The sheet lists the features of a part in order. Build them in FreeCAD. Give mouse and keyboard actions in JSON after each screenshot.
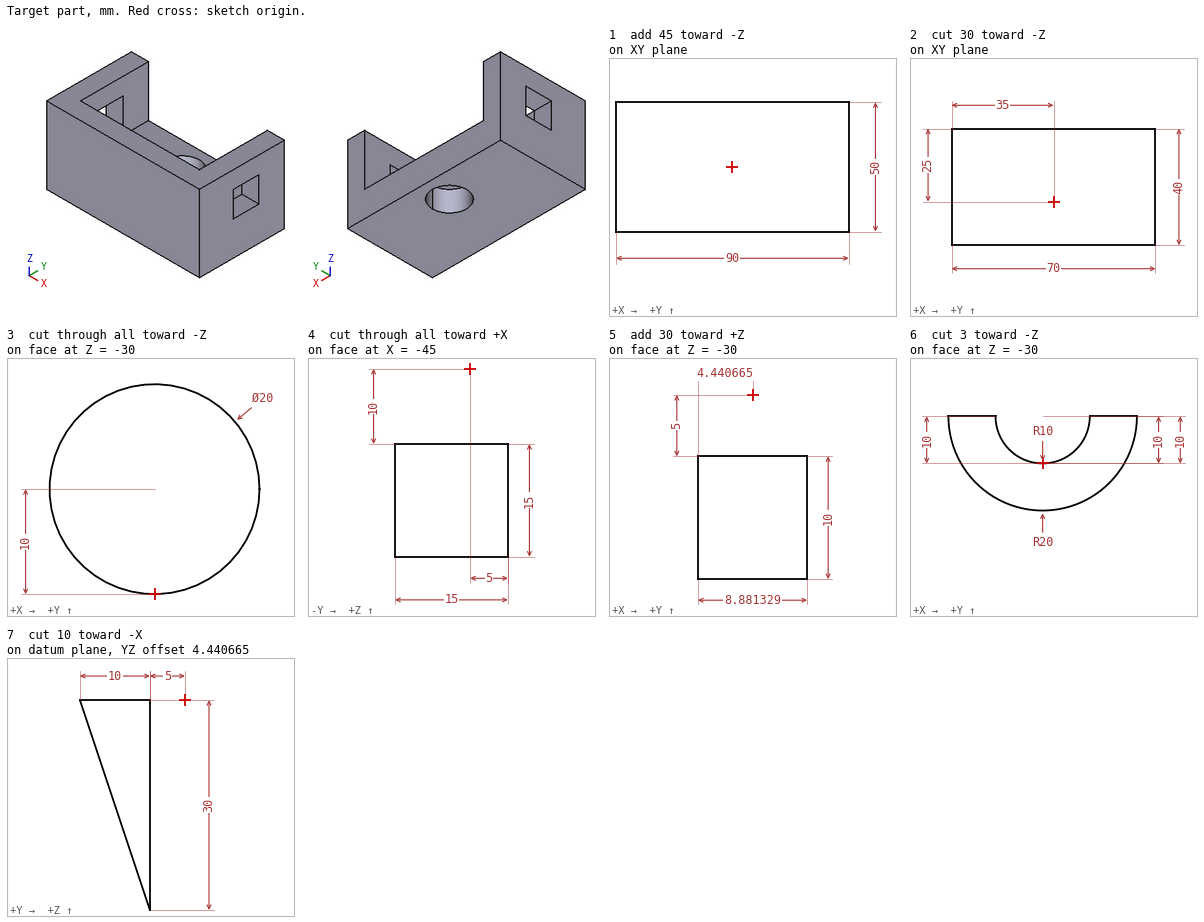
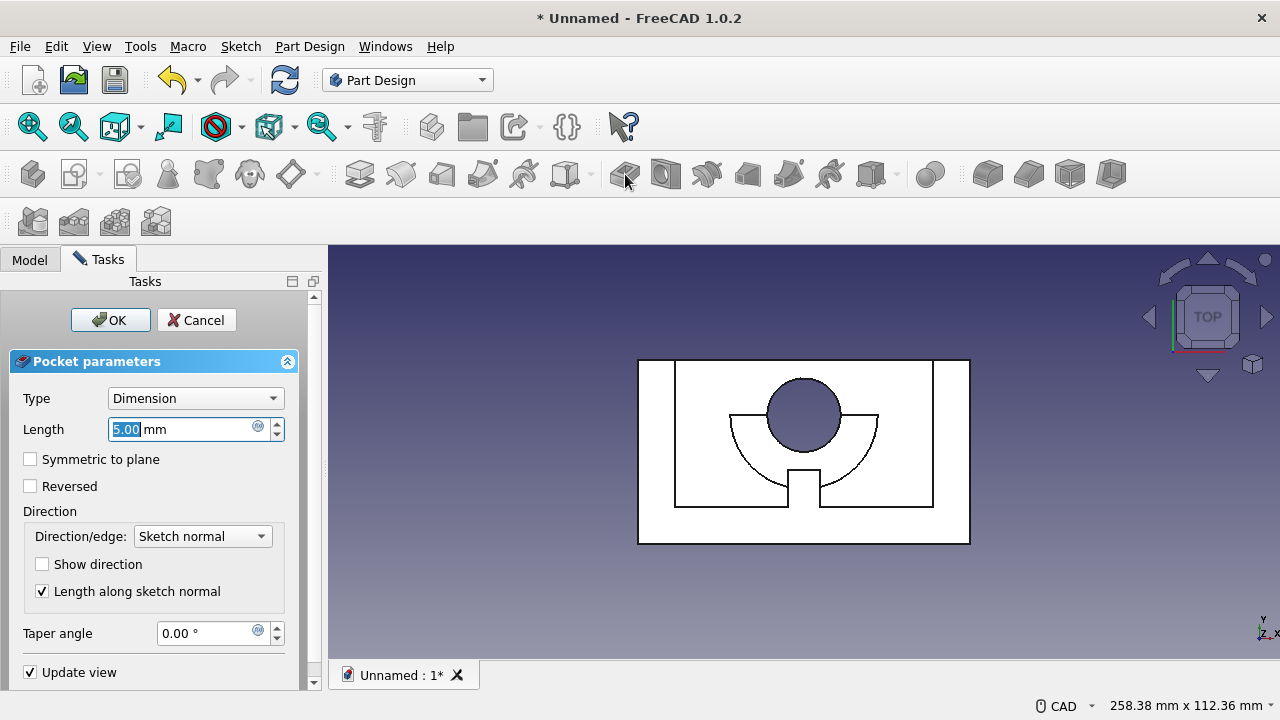
{"action": "type", "text": "3"}
{"action": "key", "text": "Tab"}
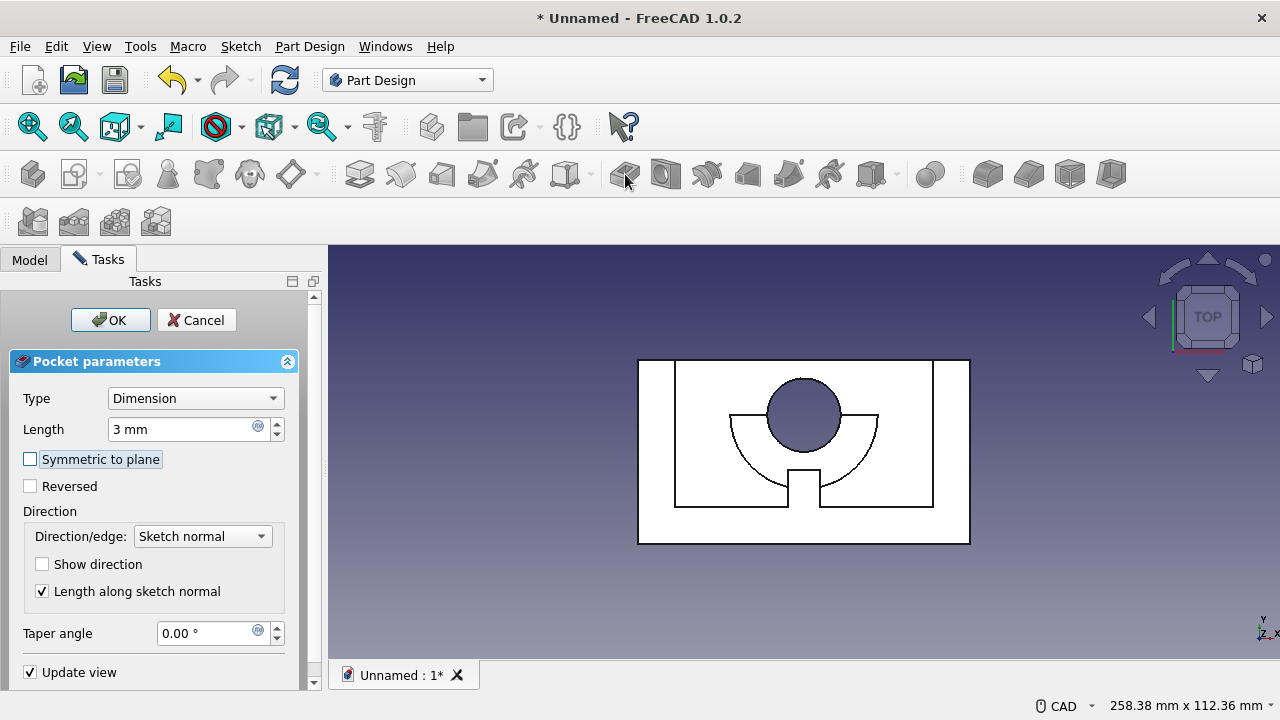
{"action": "left_click", "coordinate": [111, 320]}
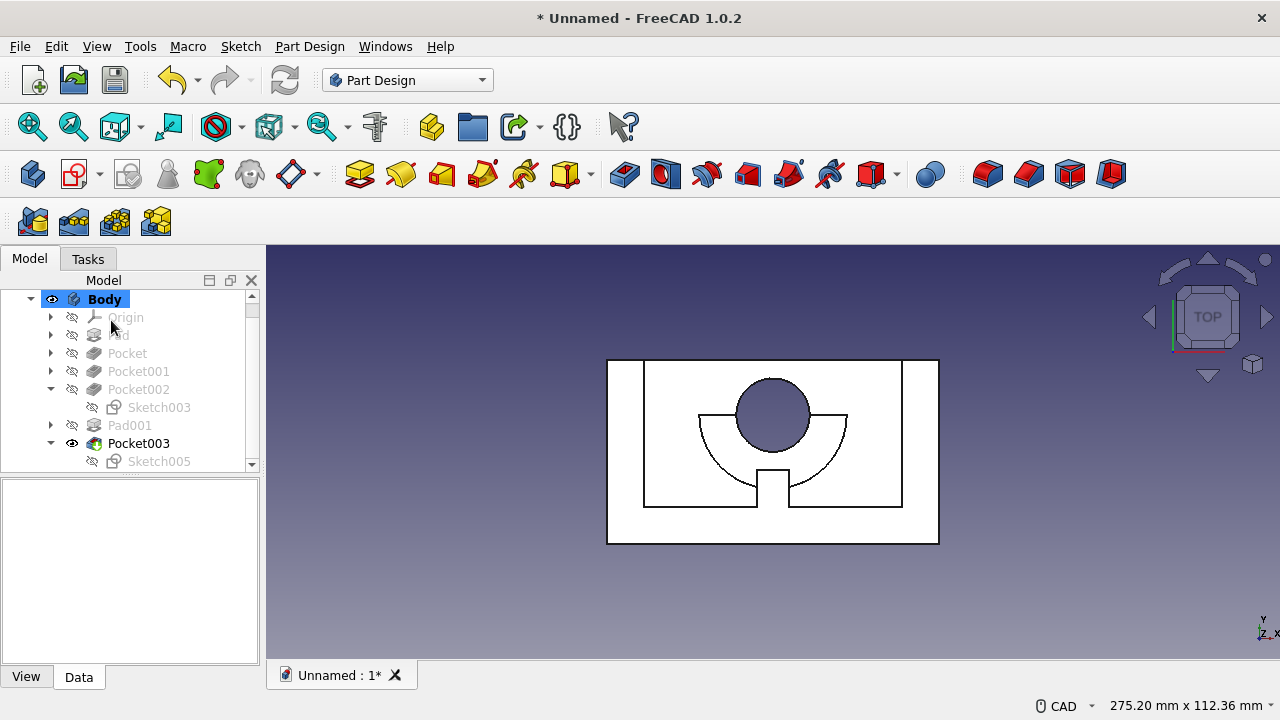
{"action": "left_click", "coordinate": [33, 128]}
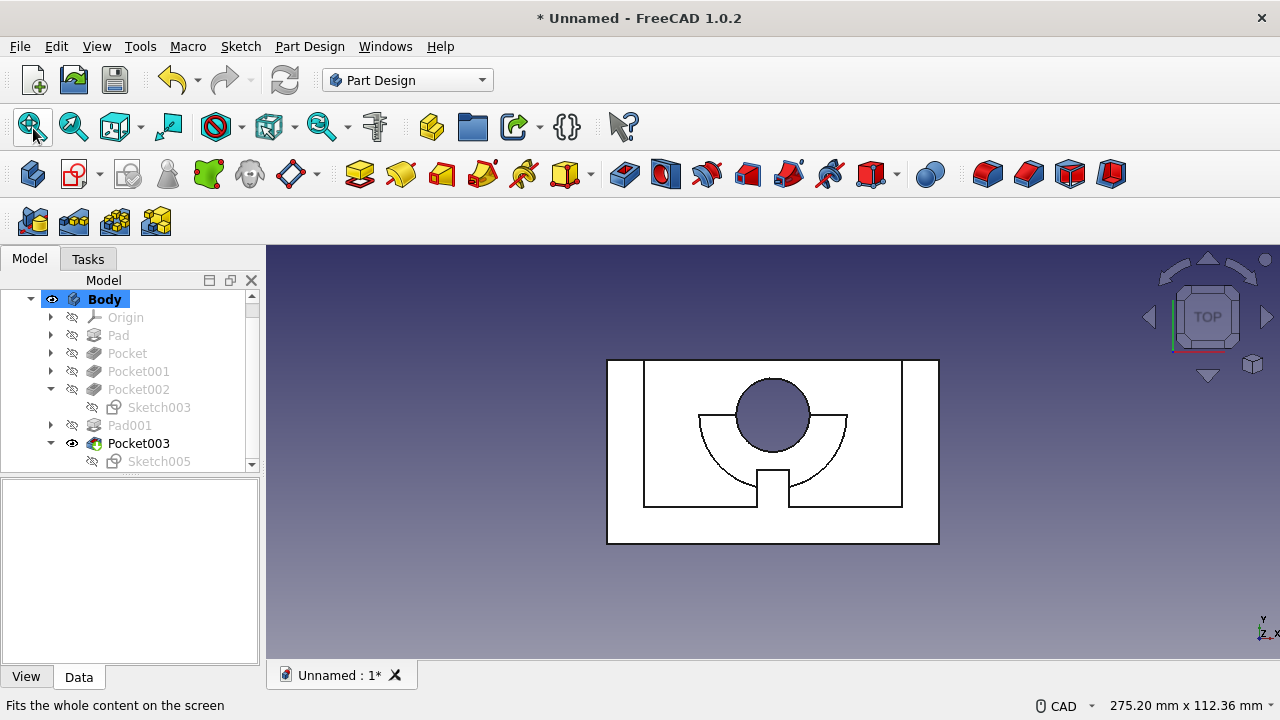
{"action": "left_click", "coordinate": [51, 317]}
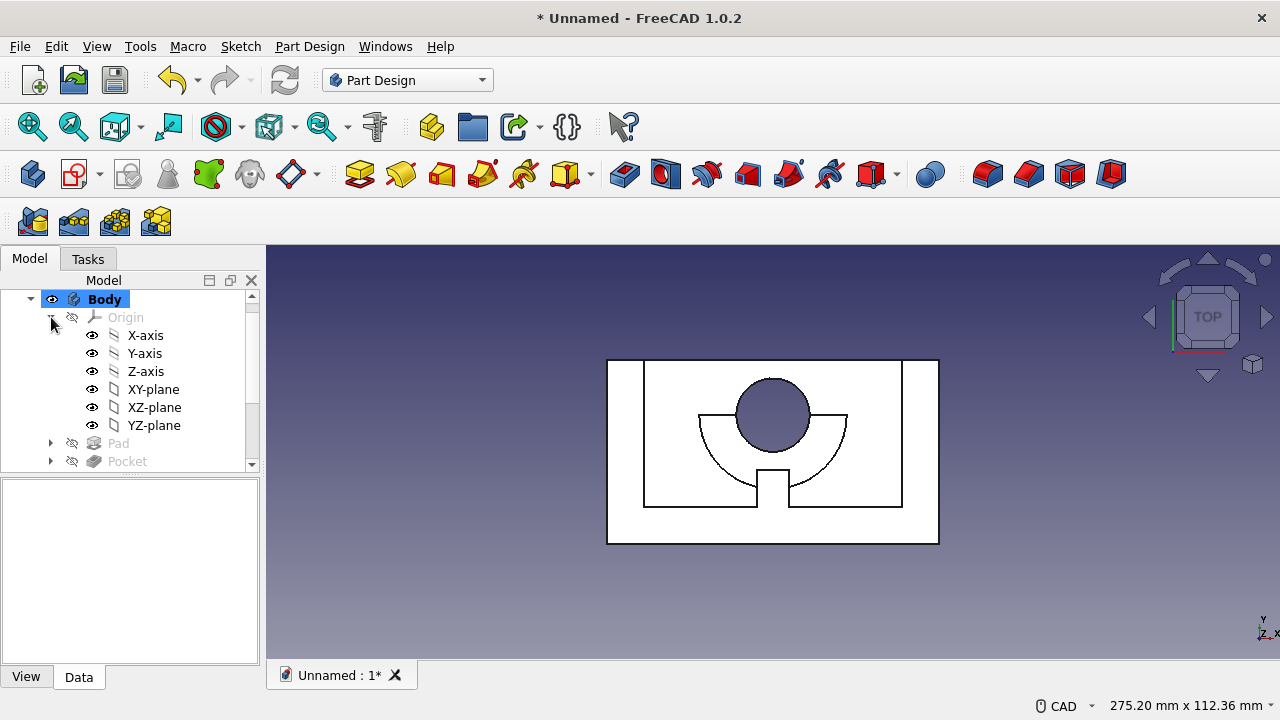
{"action": "left_click", "coordinate": [137, 425]}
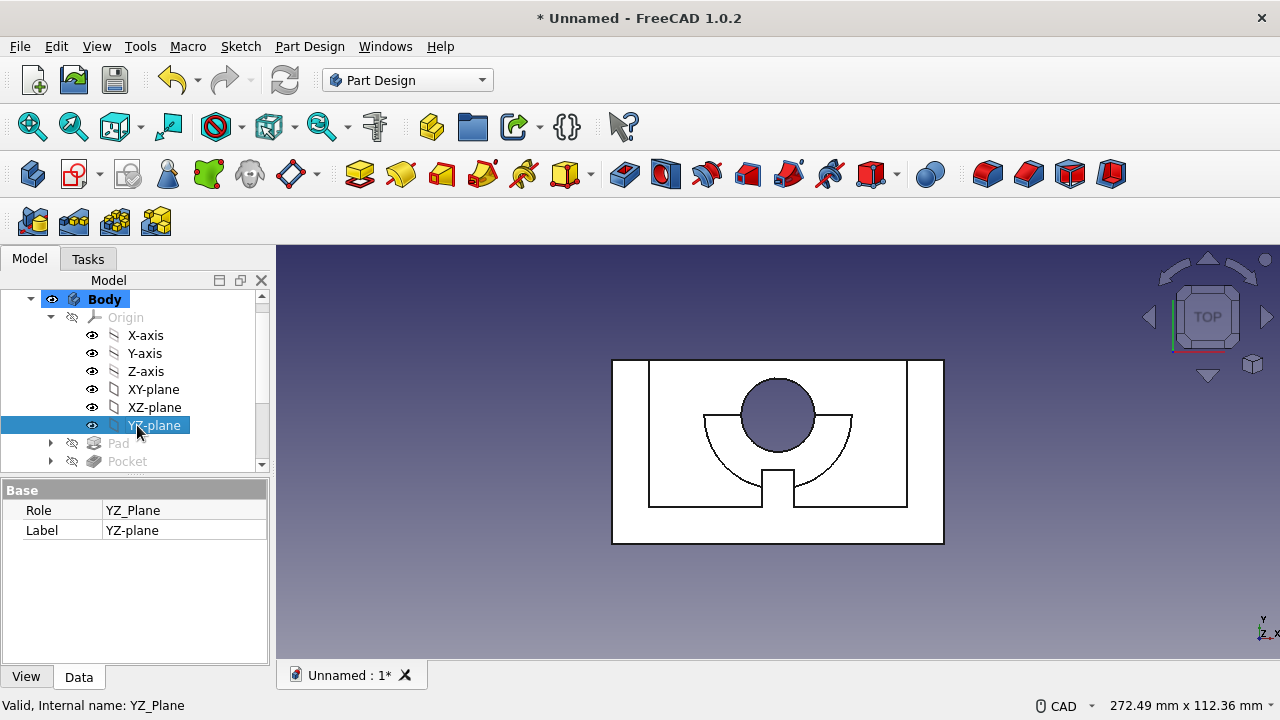
{"action": "left_click", "coordinate": [290, 174]}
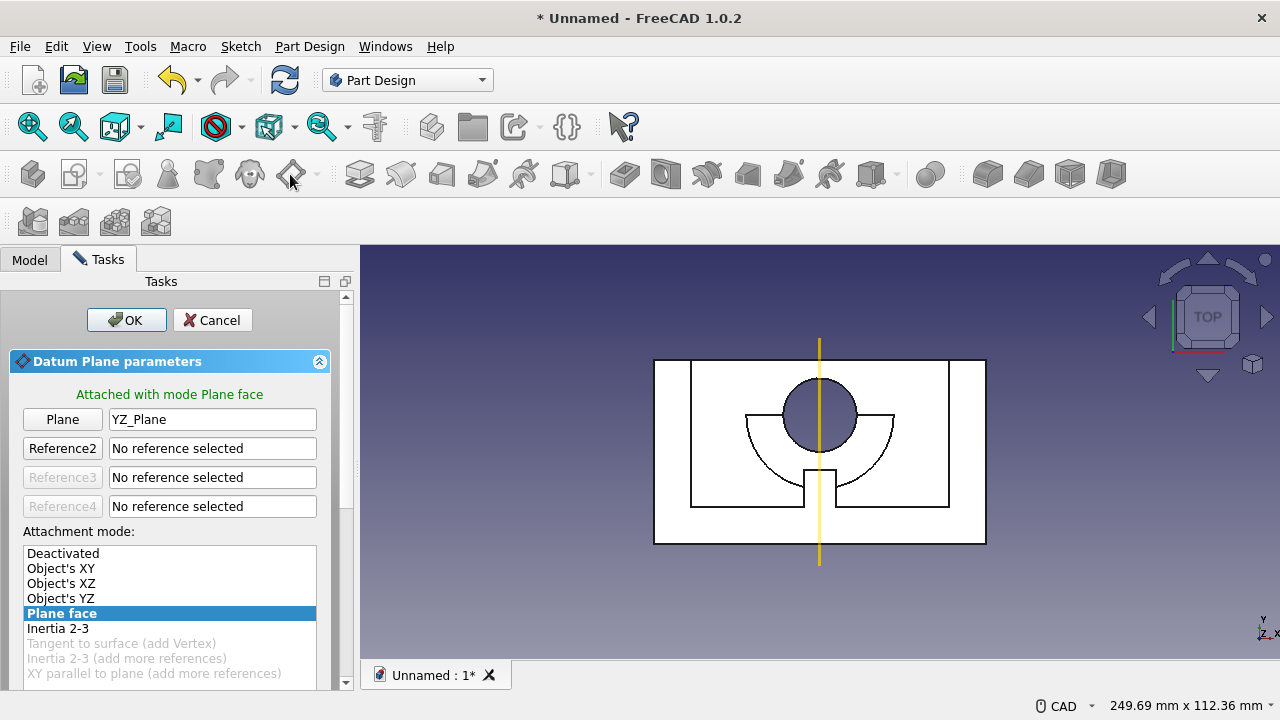
{"action": "scroll", "coordinate": [346, 490], "scroll_direction": "down", "scroll_amount": 4}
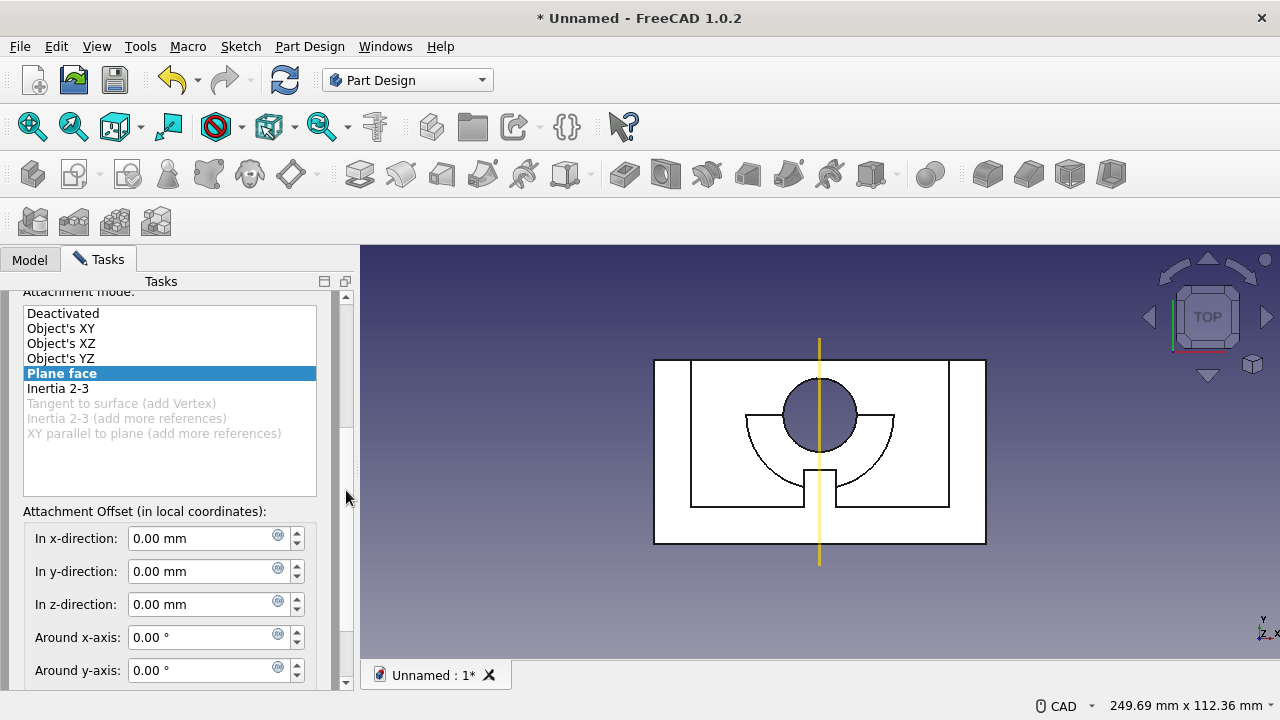
{"action": "triple_click", "coordinate": [210, 604]}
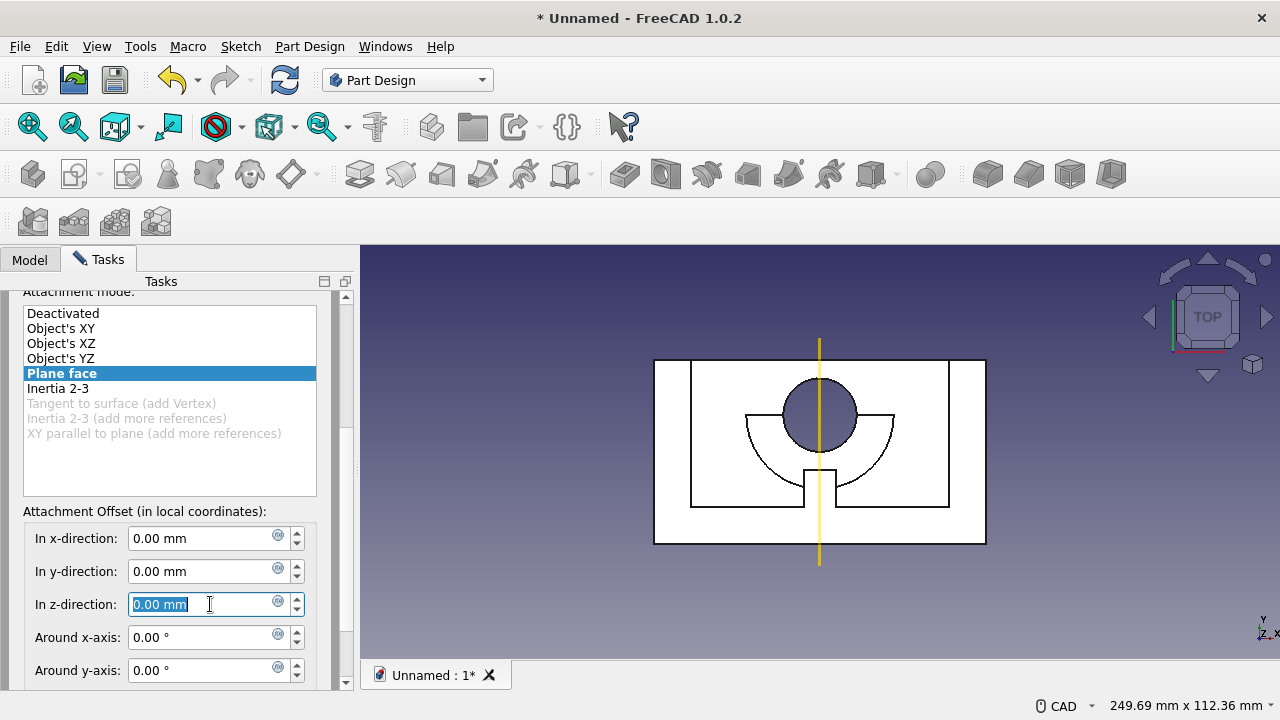
{"action": "type", "text": "4.440665"}
{"action": "key", "text": "Tab"}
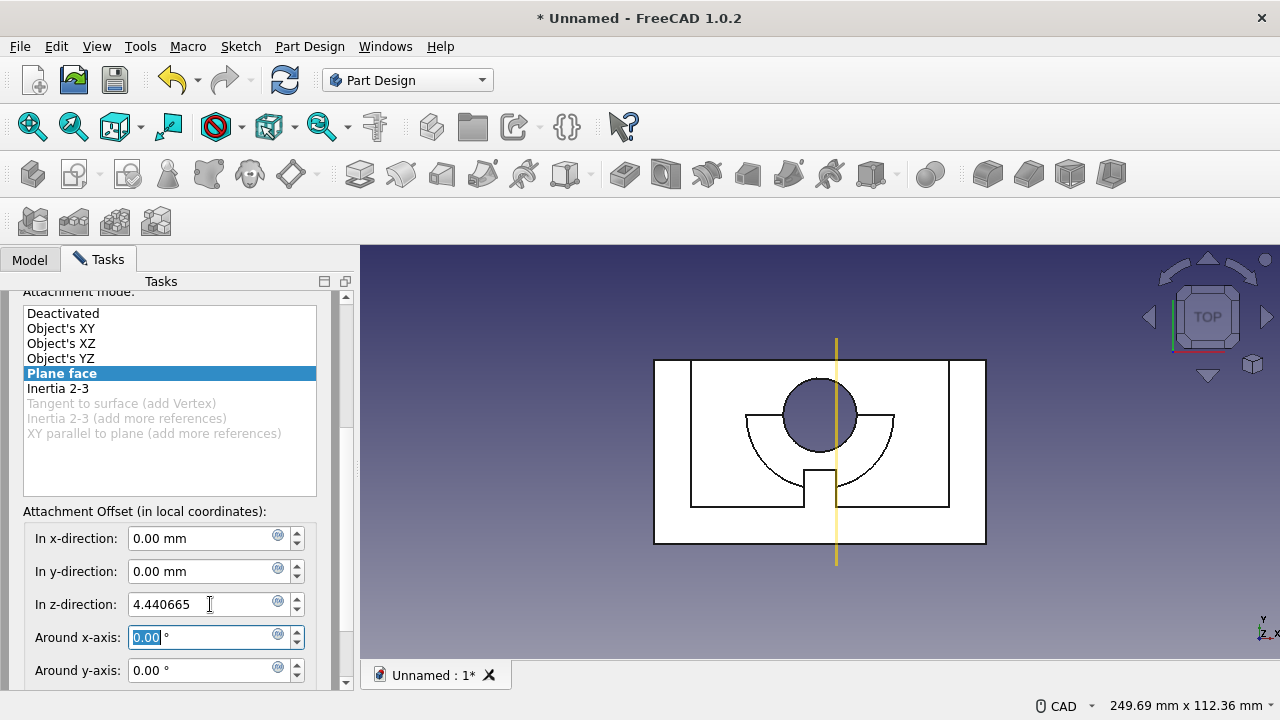
{"action": "scroll", "coordinate": [346, 490], "scroll_direction": "up", "scroll_amount": 5}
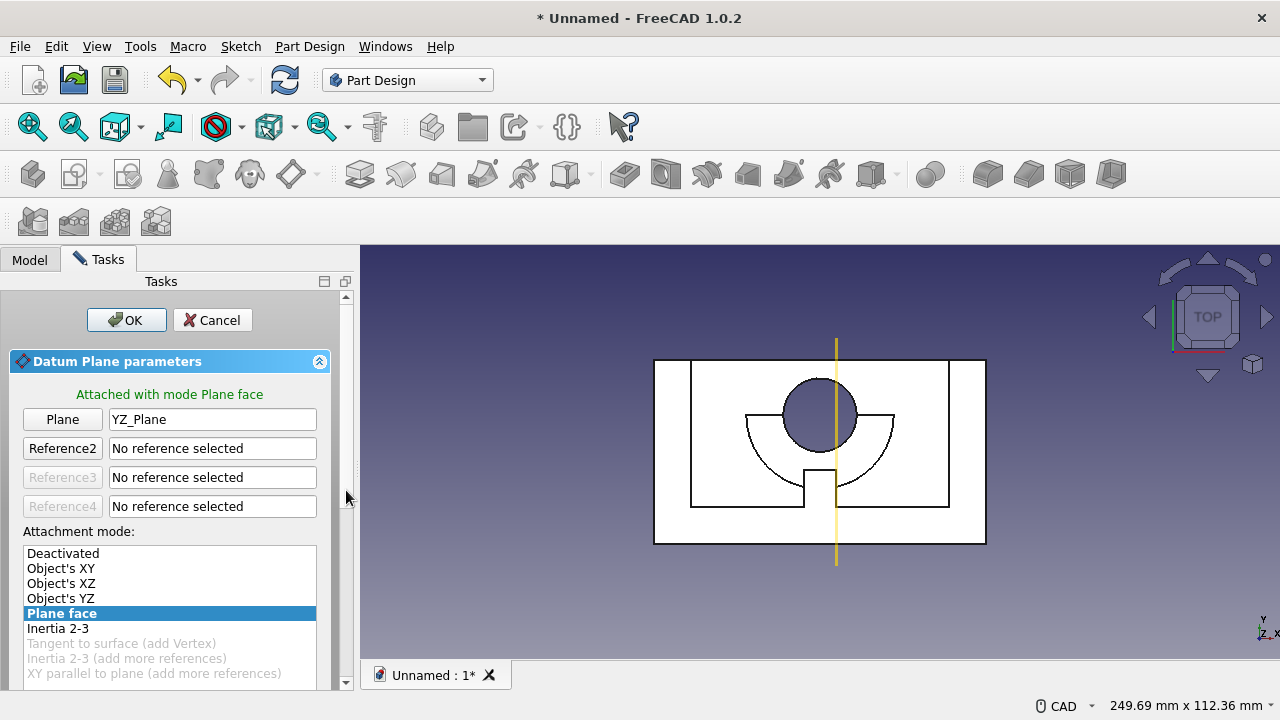
{"action": "left_click", "coordinate": [127, 320]}